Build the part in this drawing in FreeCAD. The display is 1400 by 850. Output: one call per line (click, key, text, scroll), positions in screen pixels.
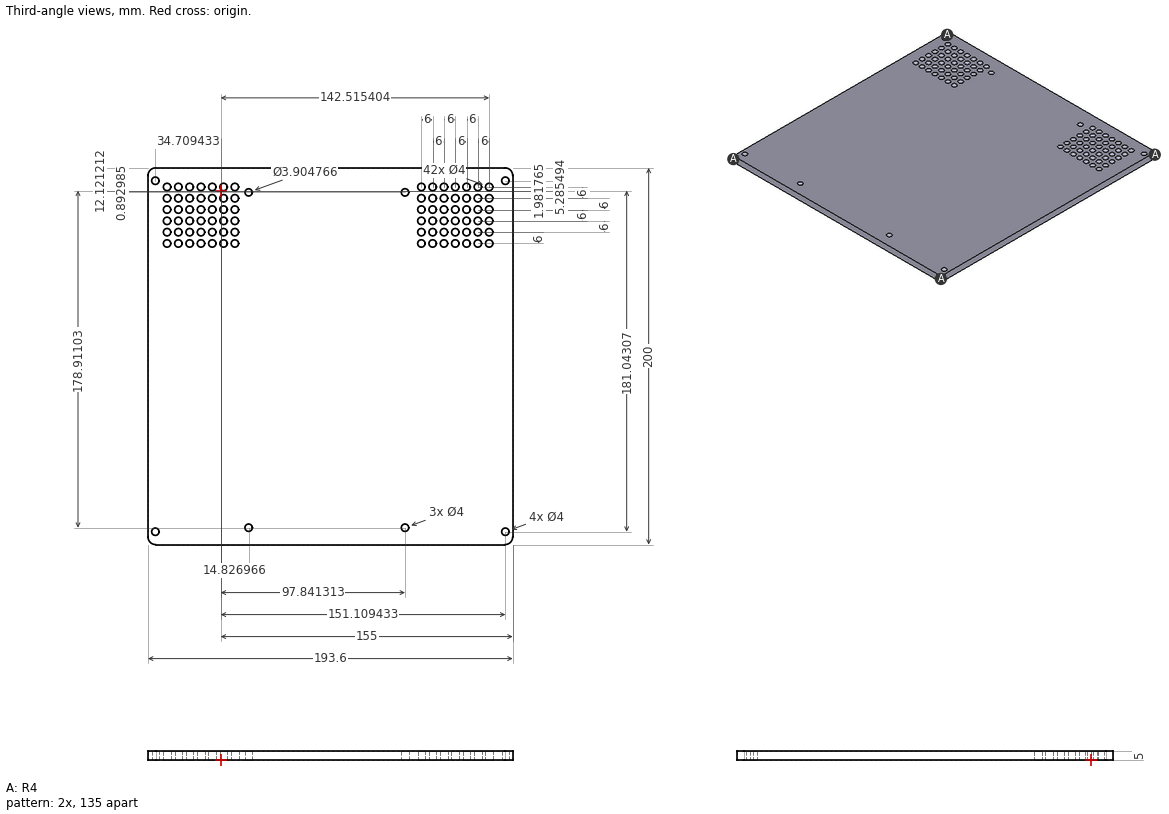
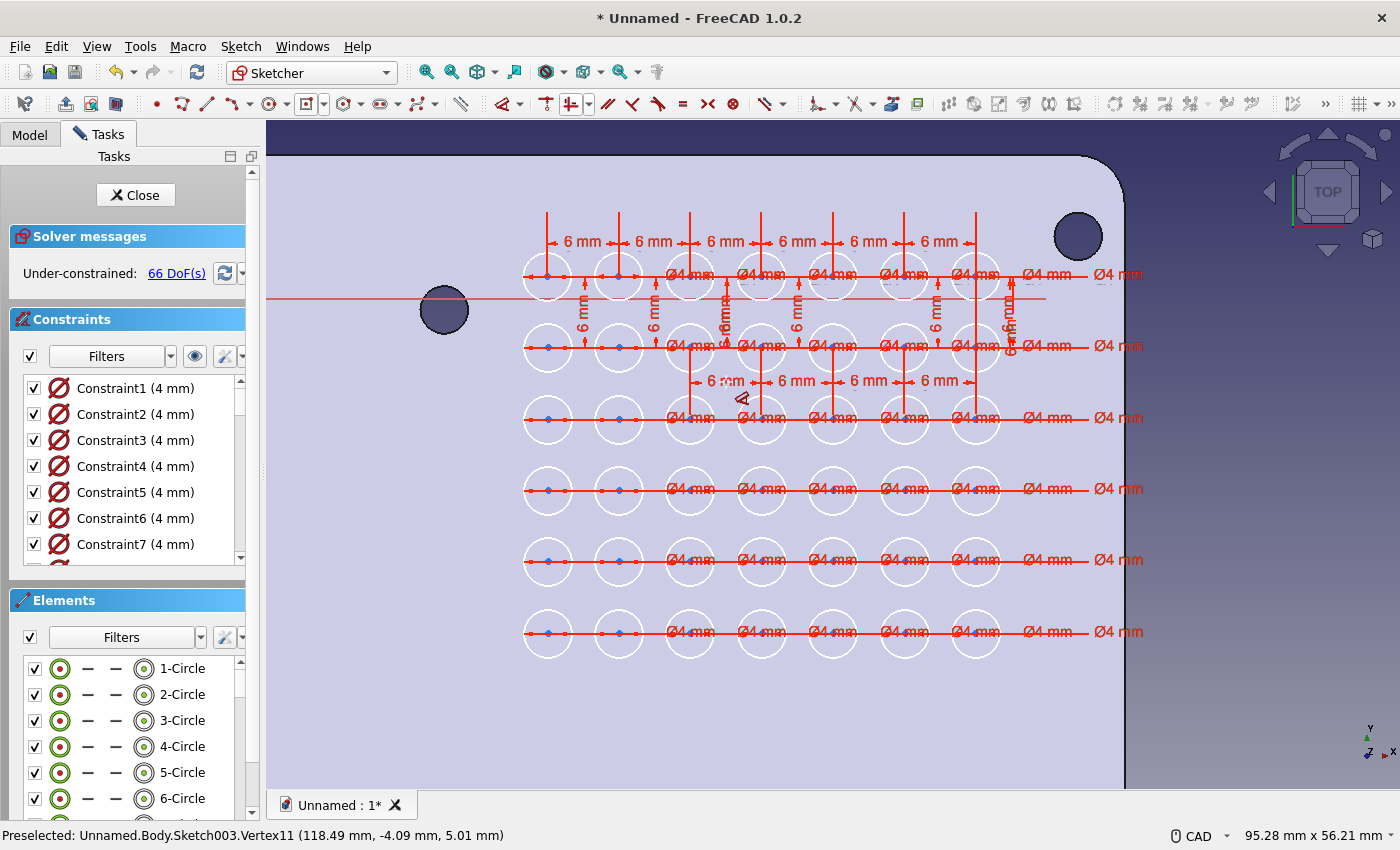
click(690, 277)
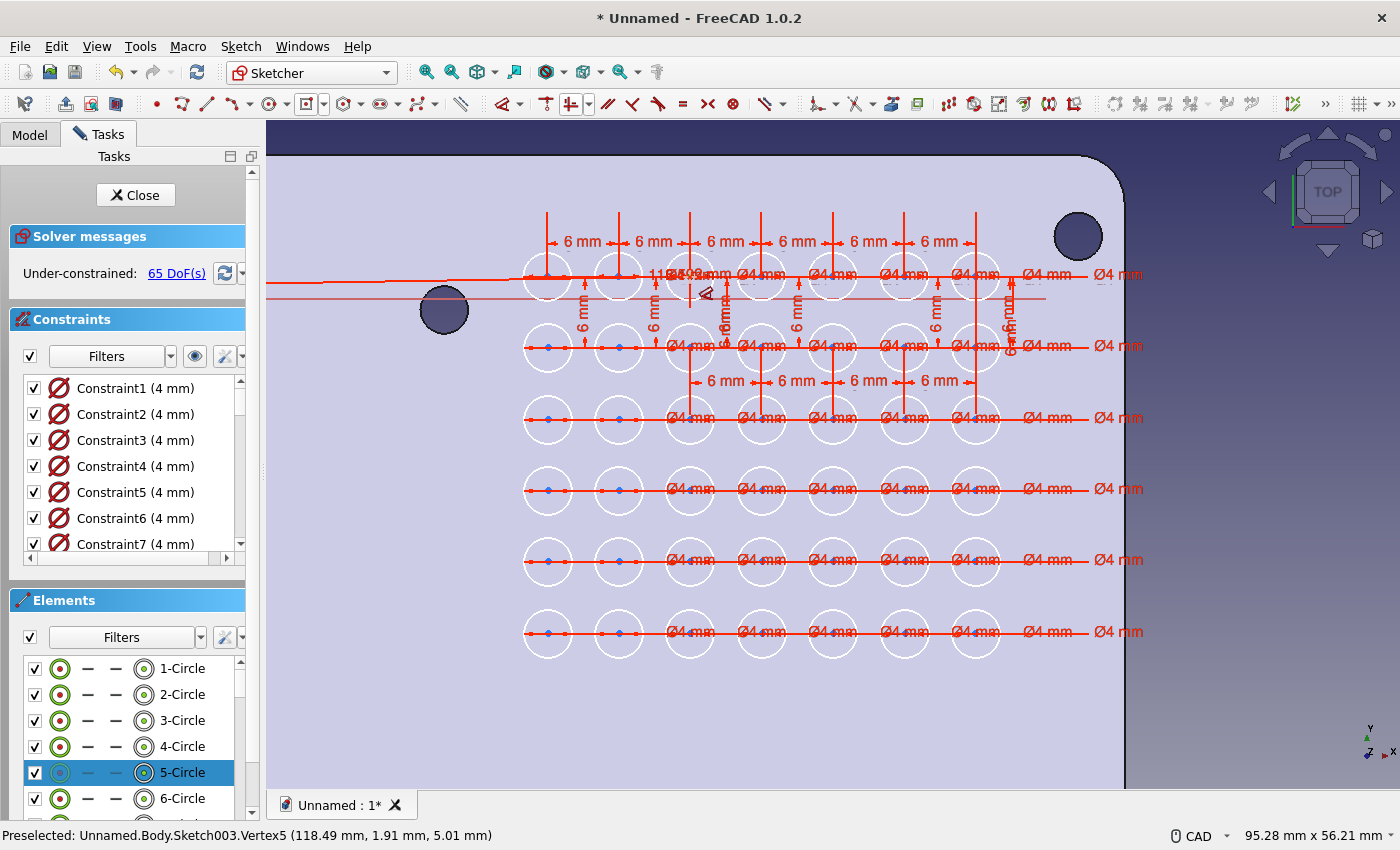
click(690, 348)
click(510, 329)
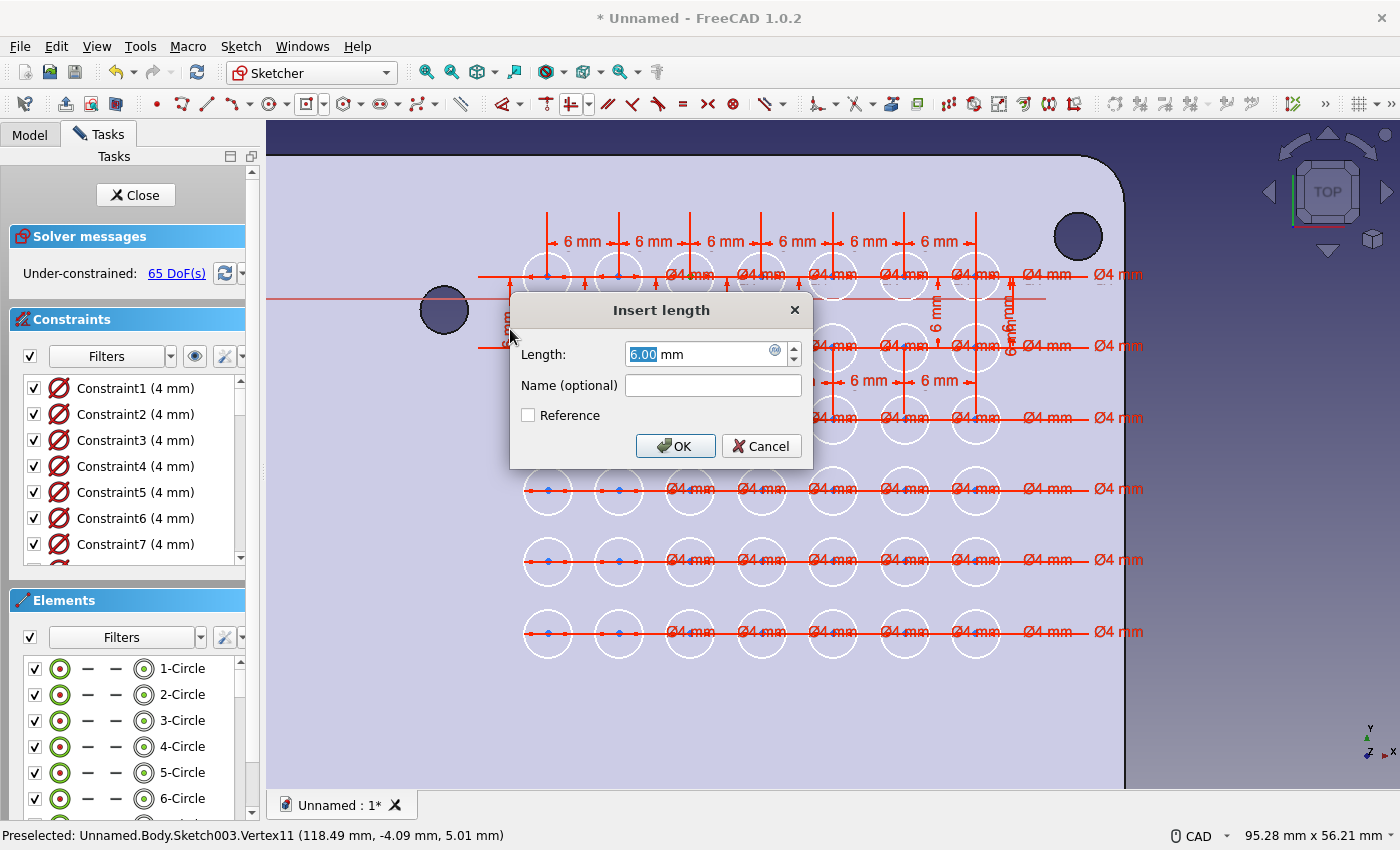
text(6)
key(Return)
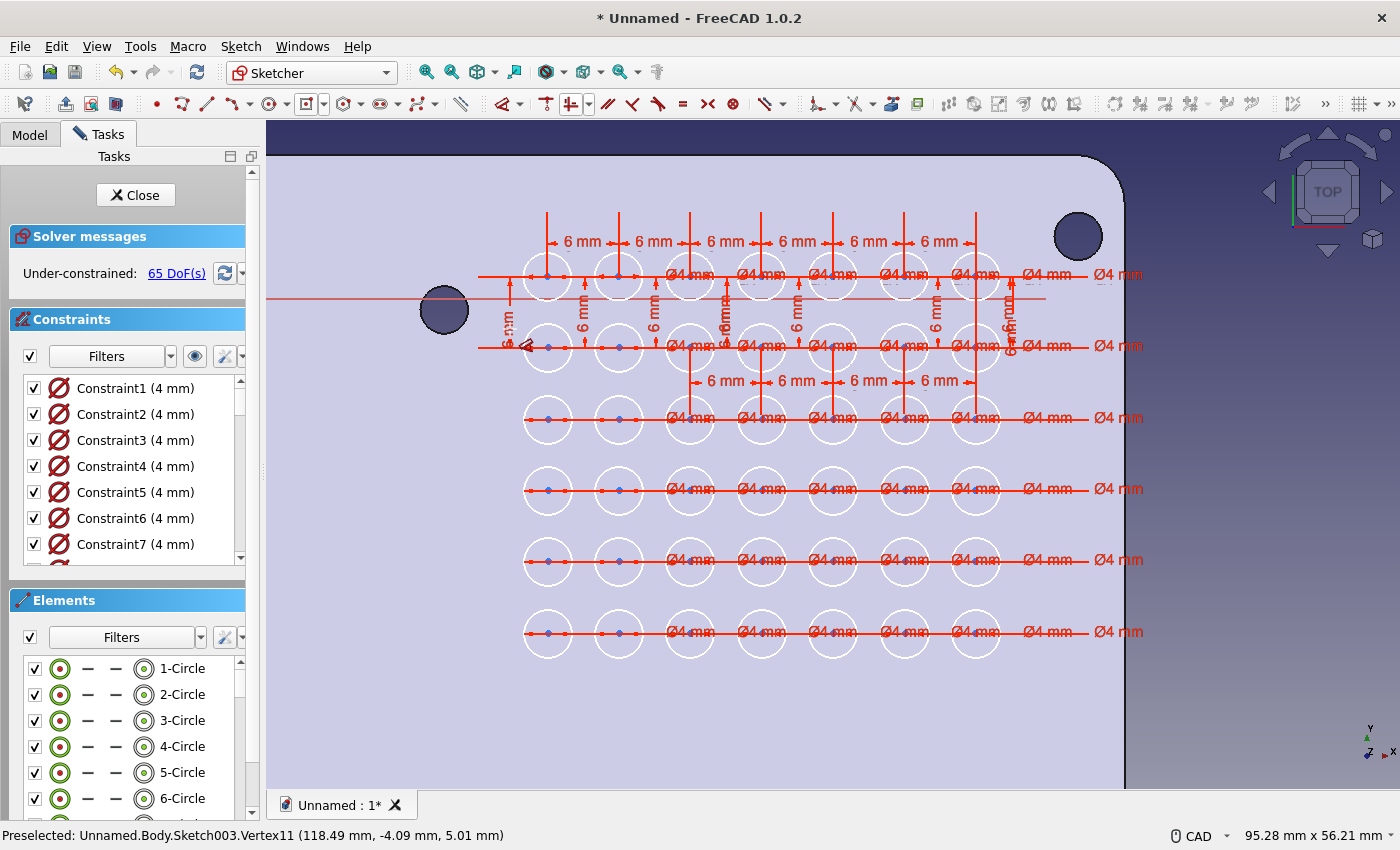
click(690, 348)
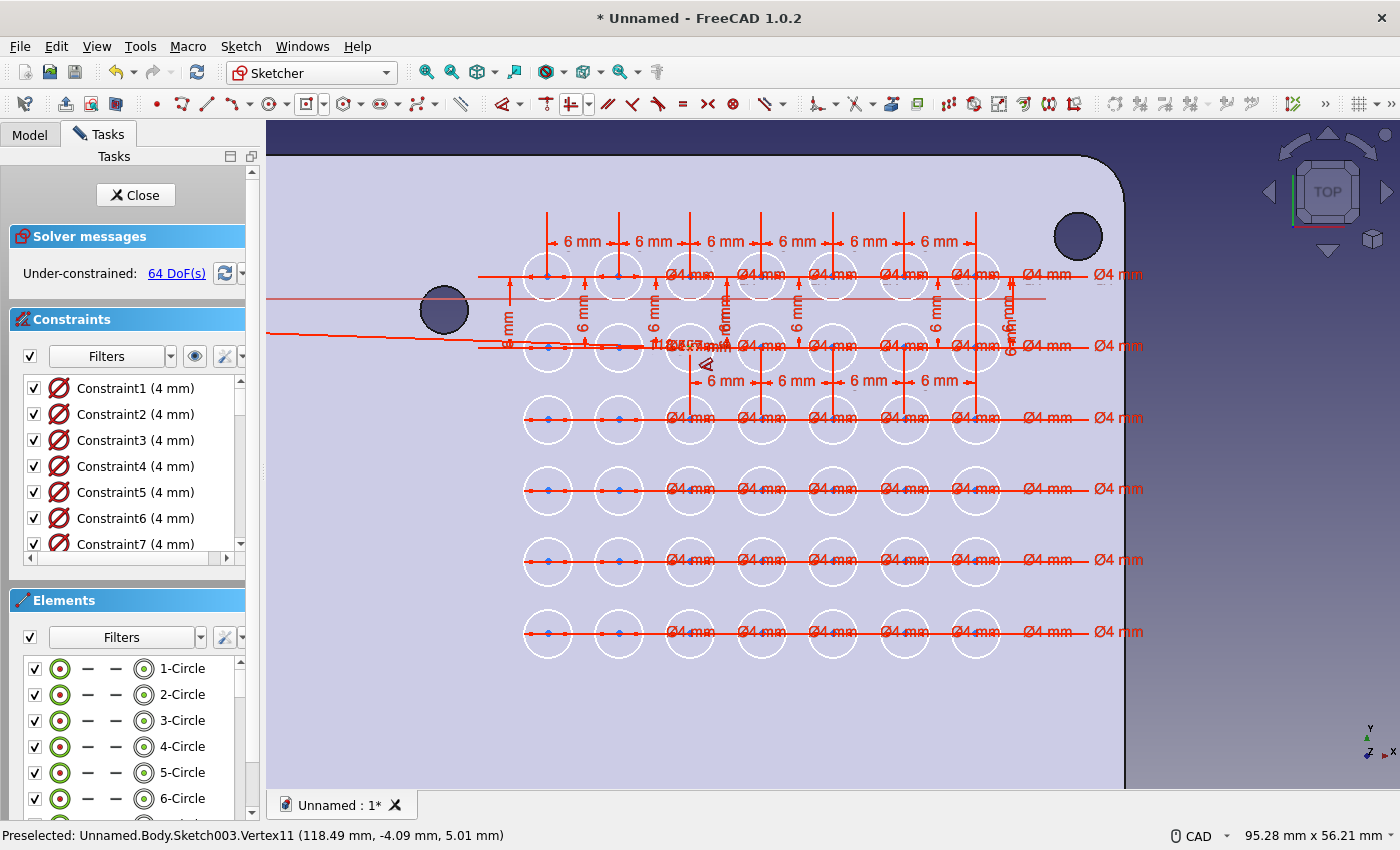
click(619, 348)
click(654, 382)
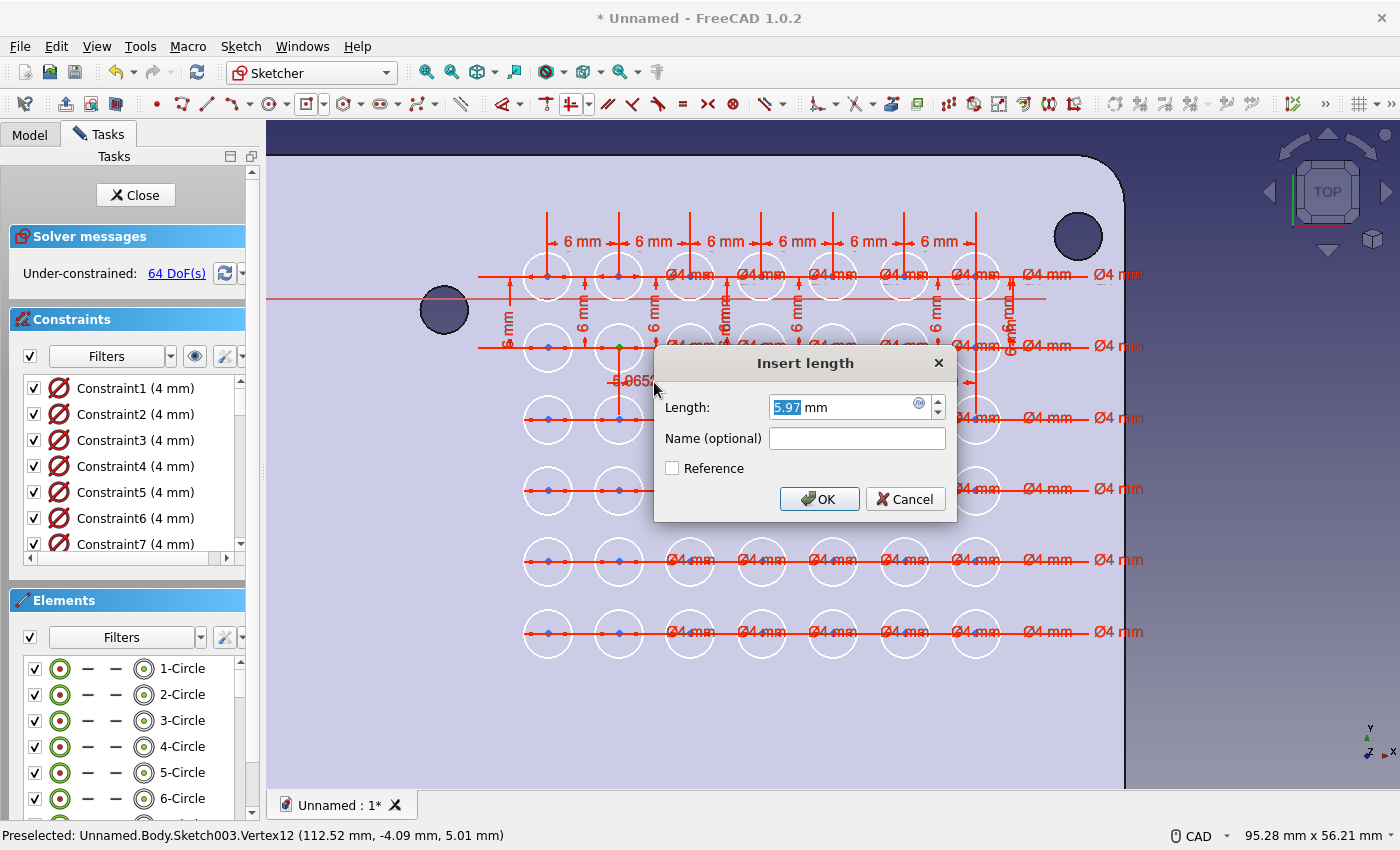
text(6)
key(Return)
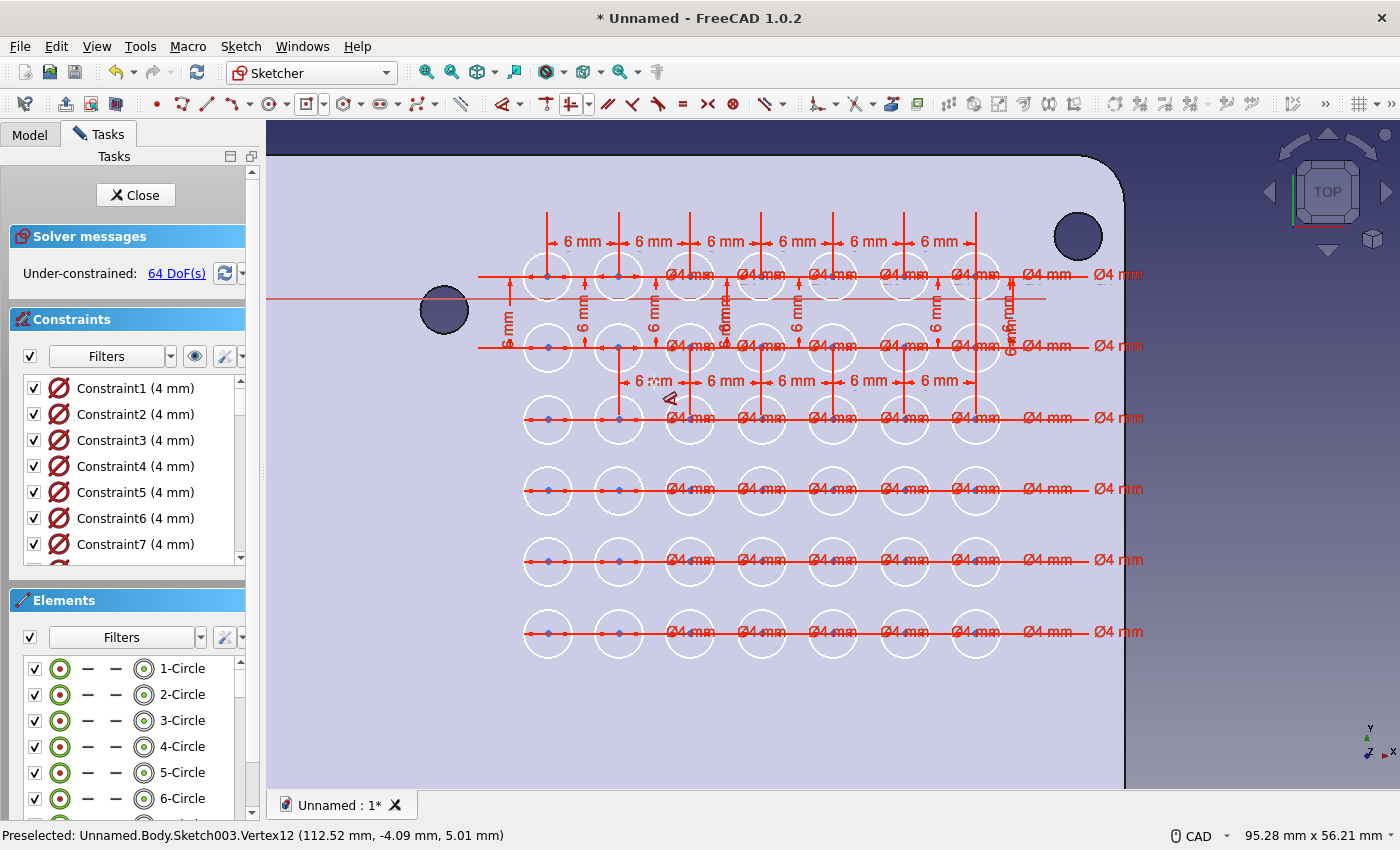
click(619, 277)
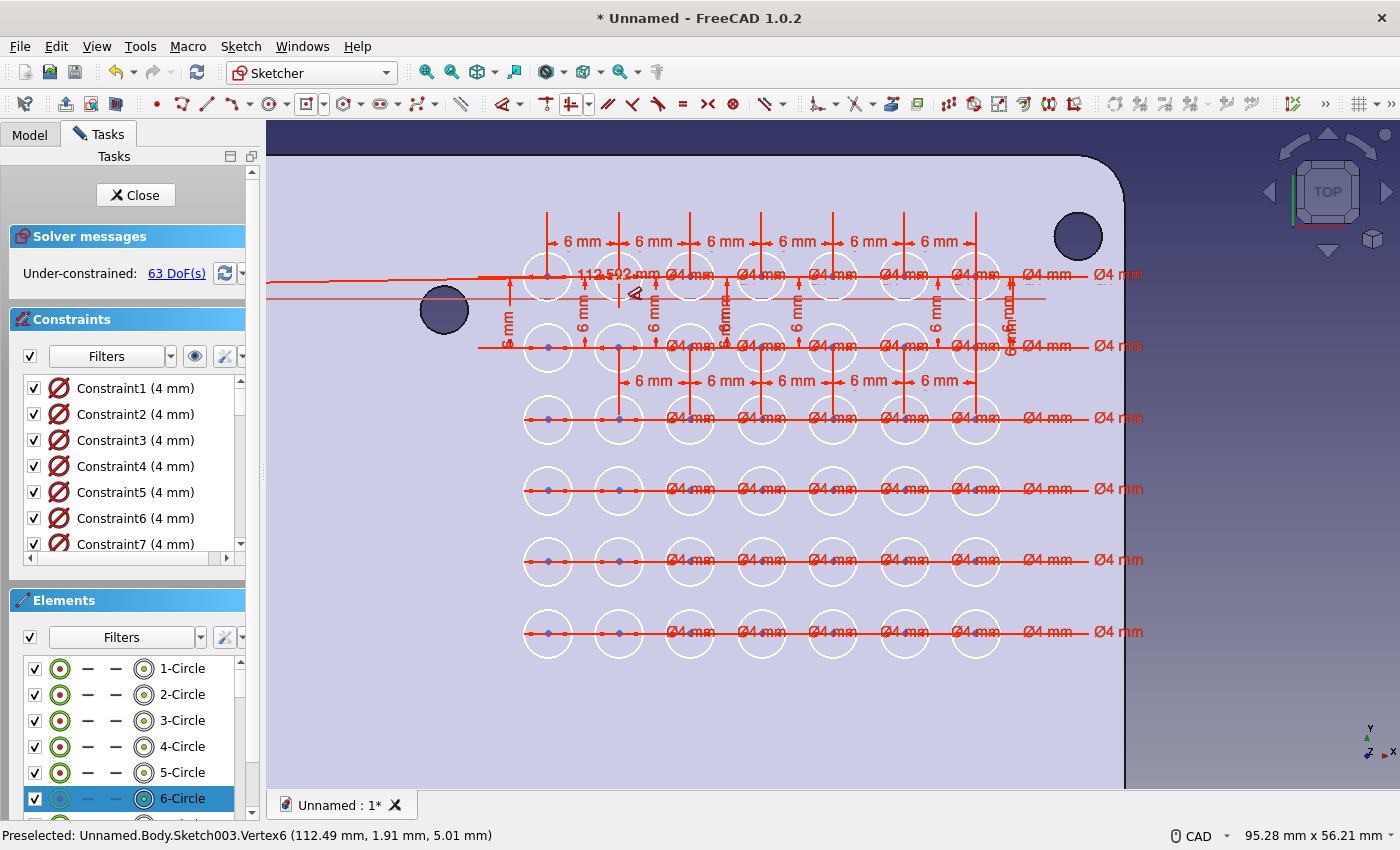
click(619, 348)
click(439, 329)